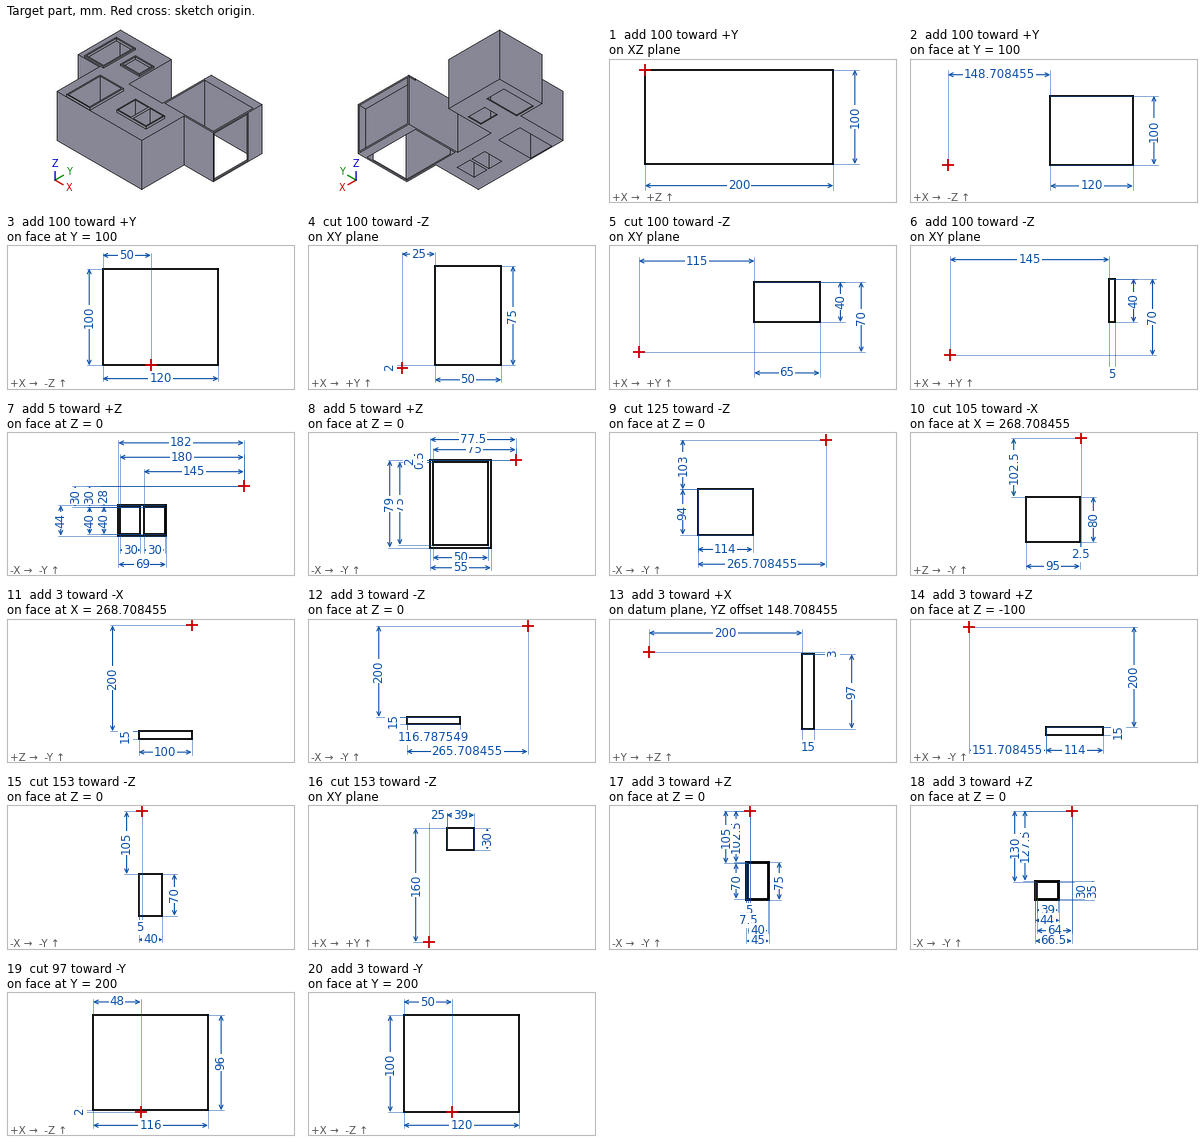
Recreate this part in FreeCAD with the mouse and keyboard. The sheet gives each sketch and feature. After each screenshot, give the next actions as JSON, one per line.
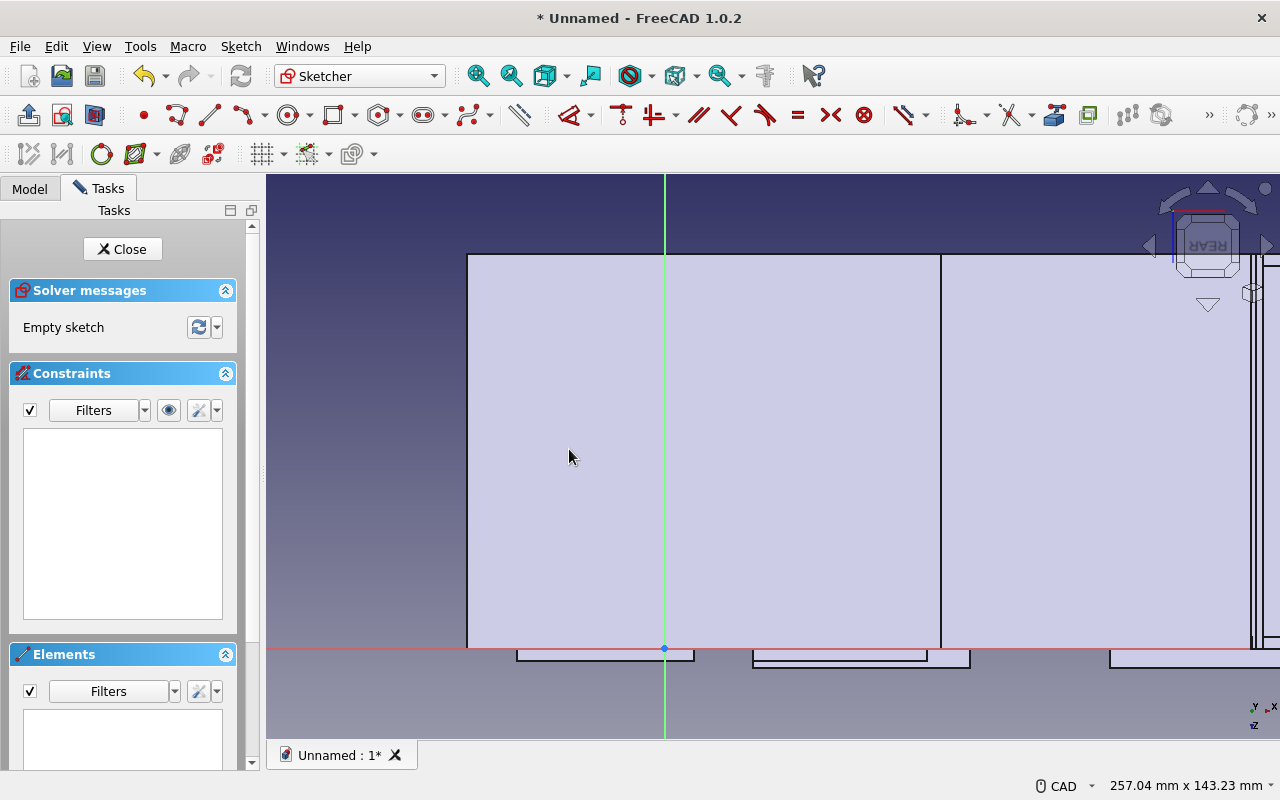
{"action": "left_click", "coordinate": [332, 116]}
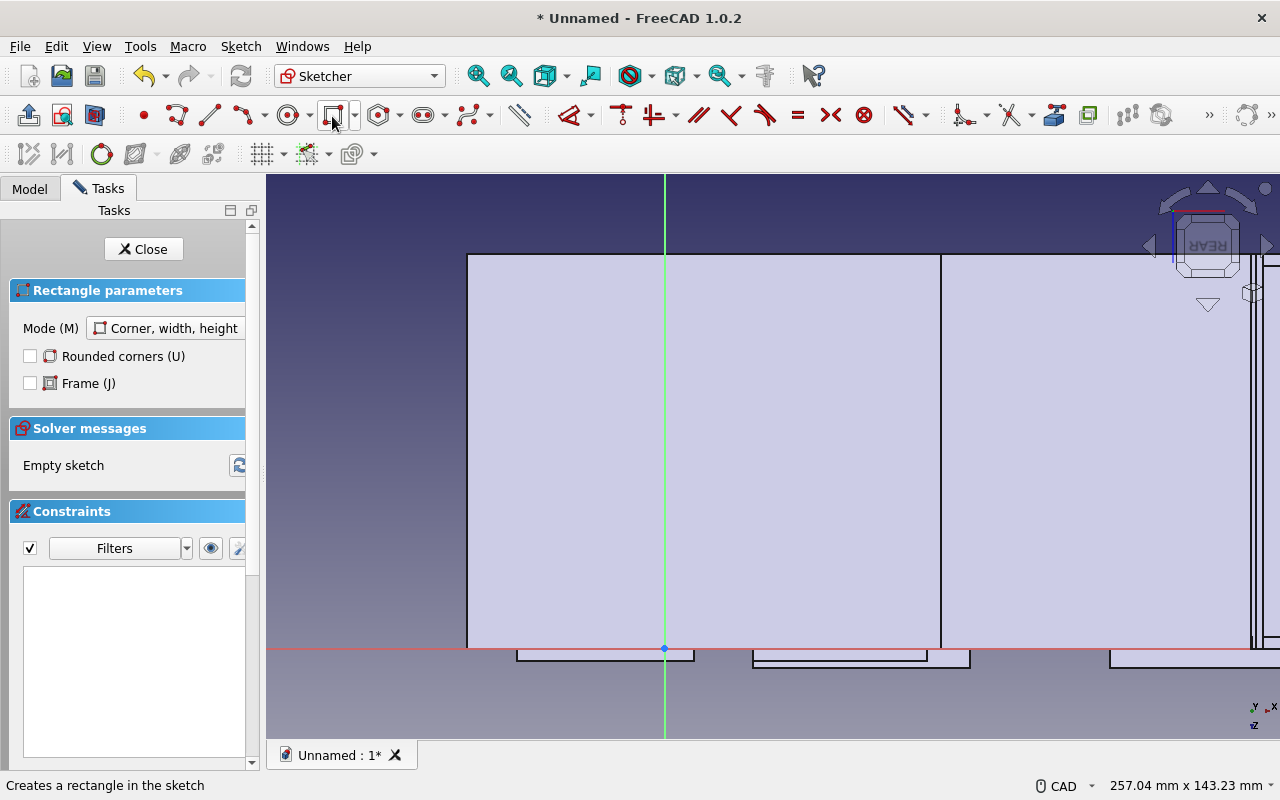
{"action": "left_click", "coordinate": [475, 262]}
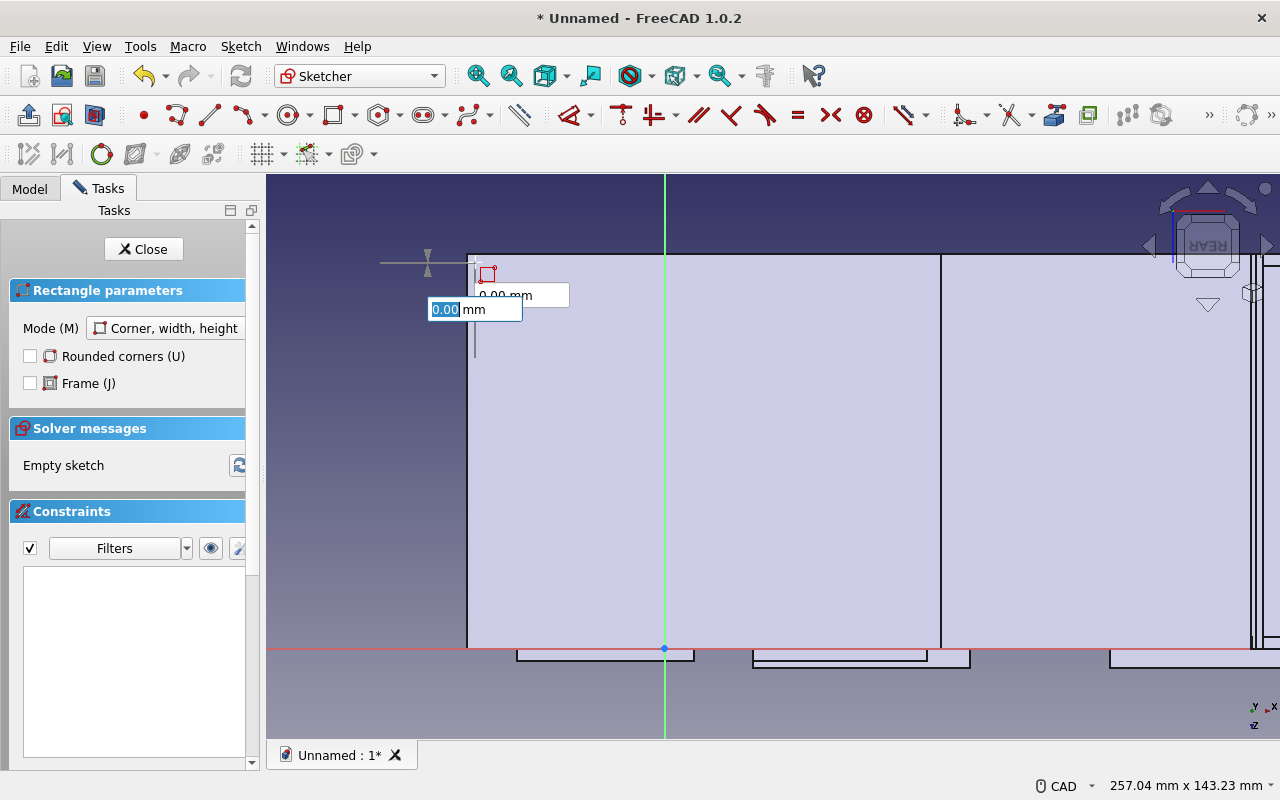
{"action": "scroll", "coordinate": [933, 641], "scroll_direction": "up", "scroll_amount": 4}
{"action": "mouse_move", "coordinate": [932, 640]}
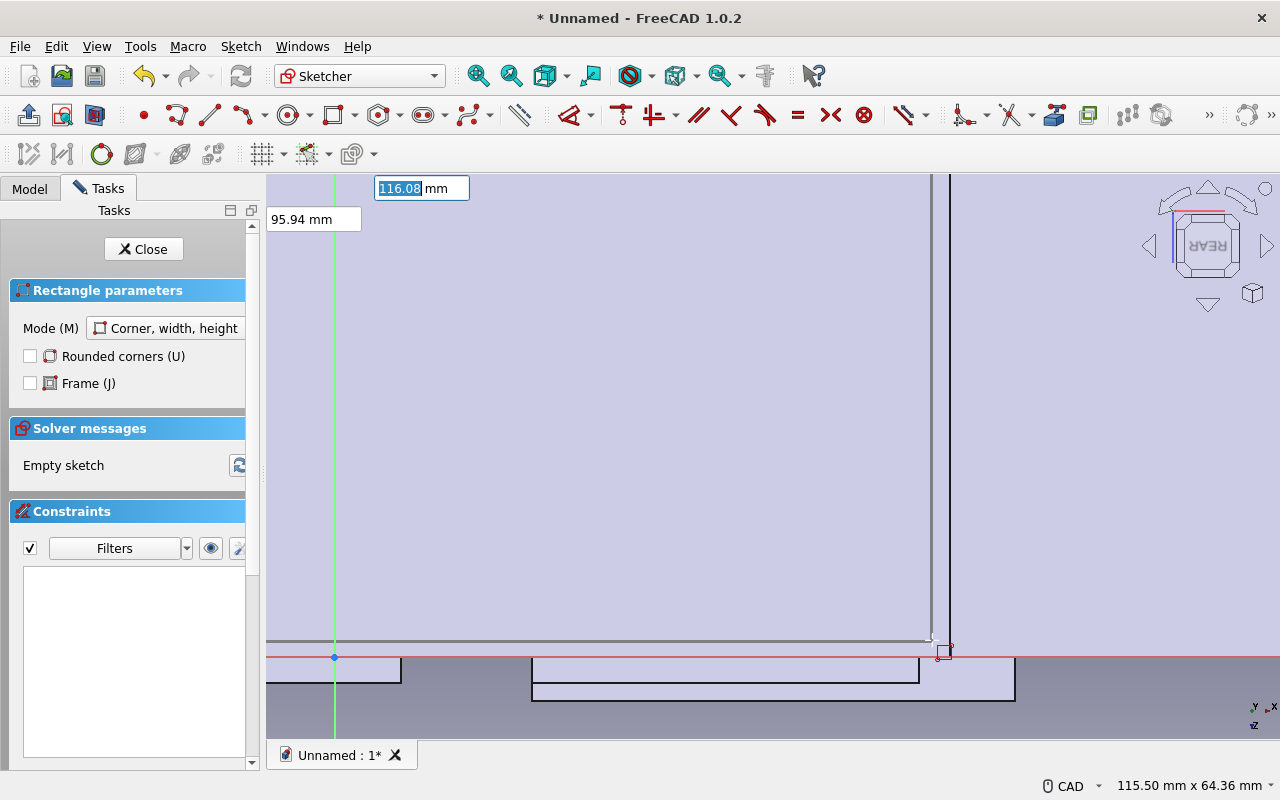
{"action": "type", "text": "116"}
{"action": "key", "text": "Tab"}
{"action": "type", "text": "96"}
{"action": "key", "text": "Return"}
{"action": "key", "text": "Escape"}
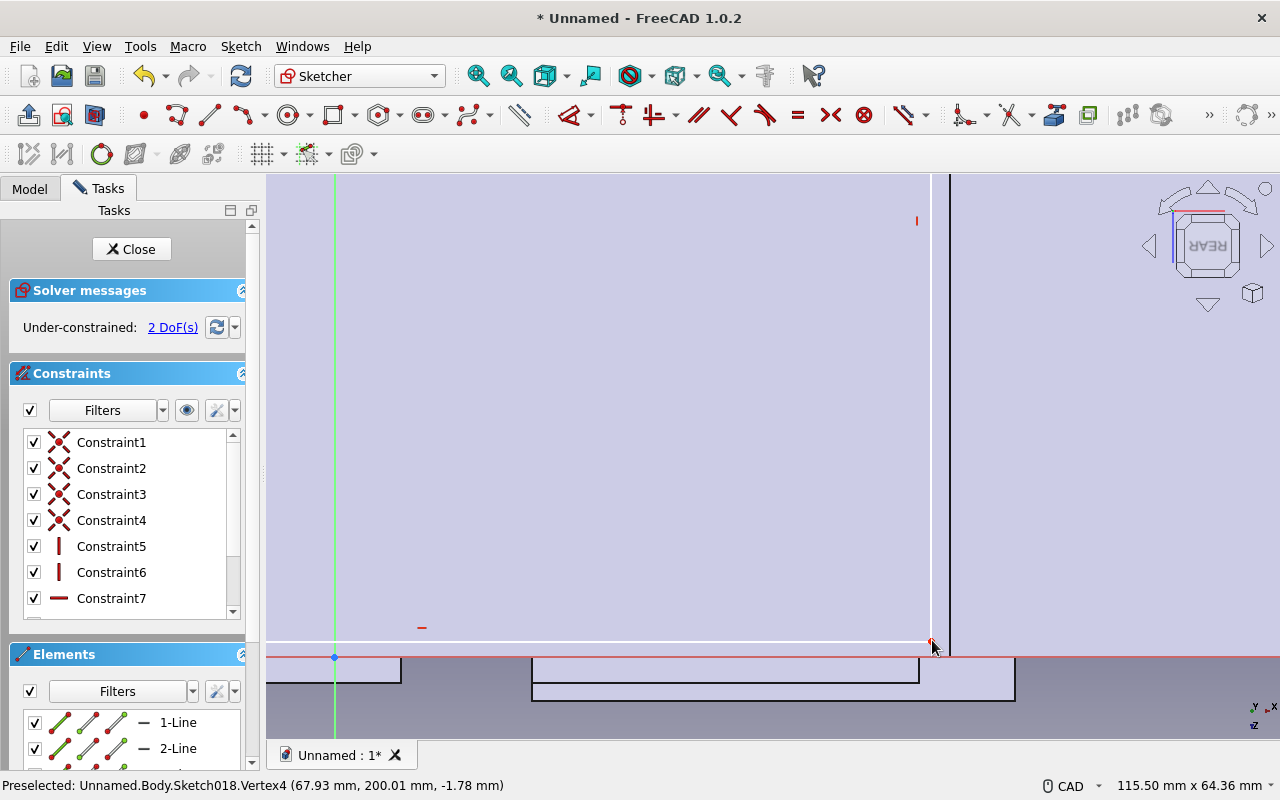
{"action": "left_click", "coordinate": [568, 116]}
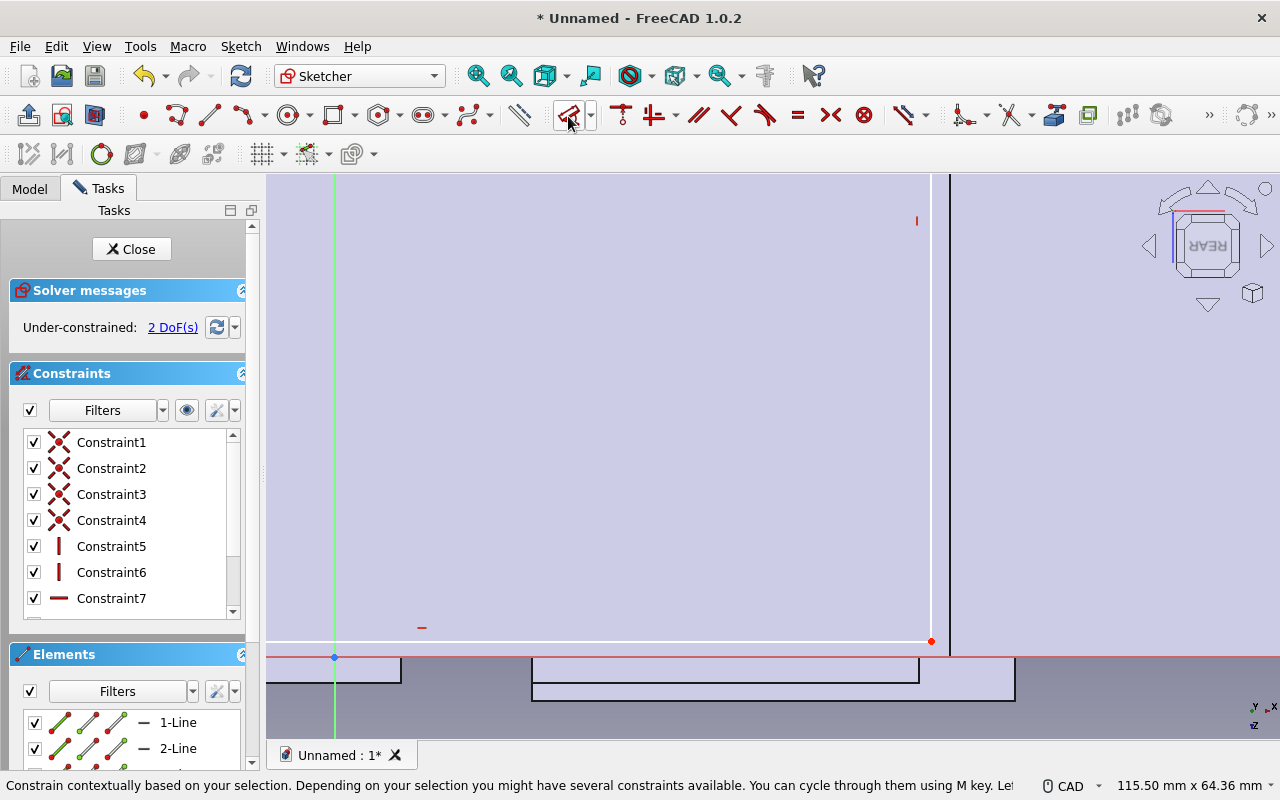
{"action": "scroll", "coordinate": [934, 644], "scroll_direction": "down", "scroll_amount": 4}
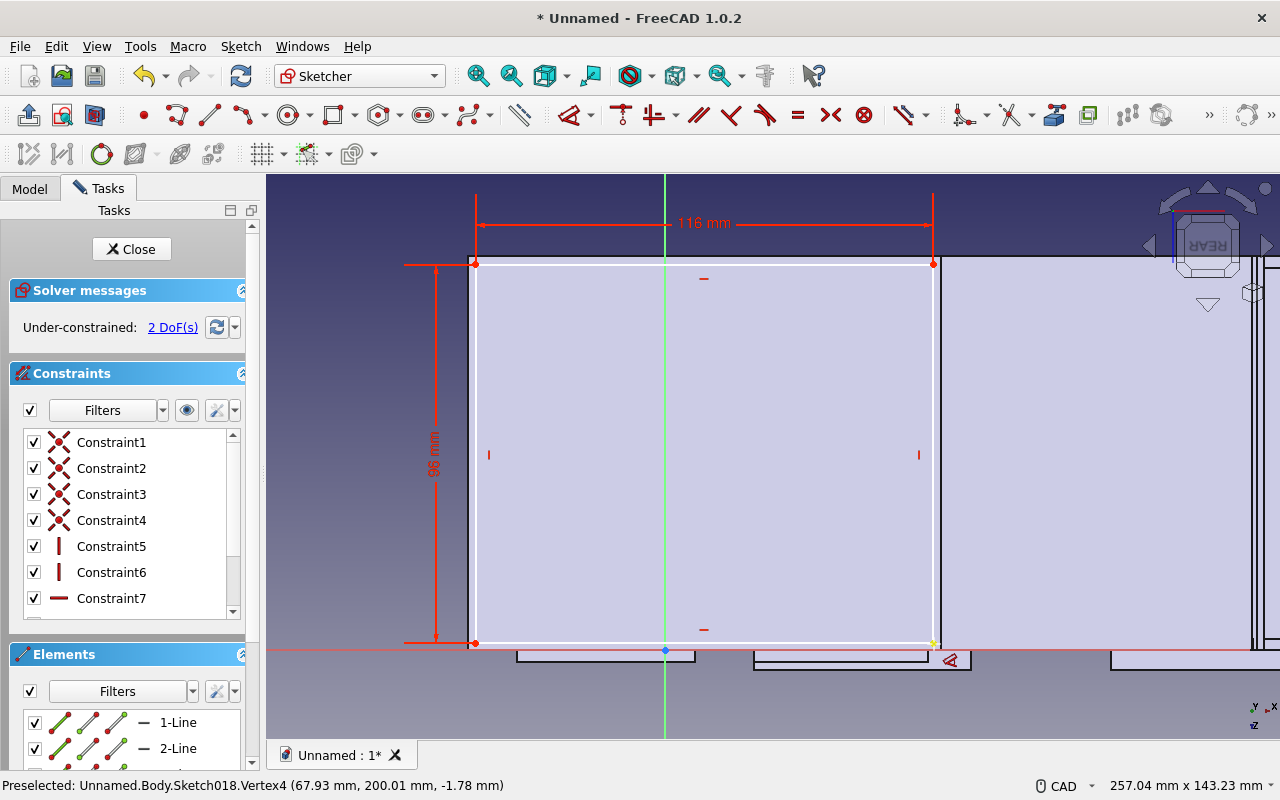
{"action": "scroll", "coordinate": [476, 643], "scroll_direction": "up", "scroll_amount": 9}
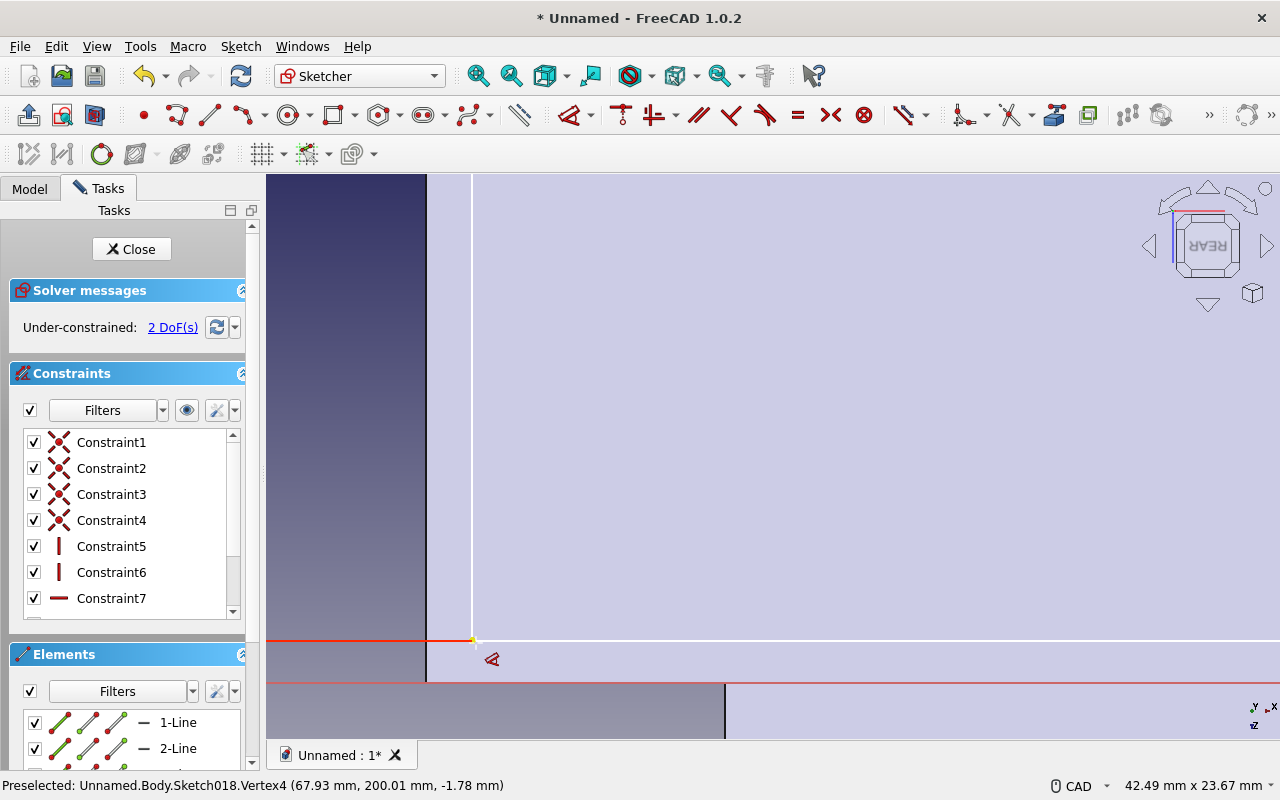
{"action": "left_click", "coordinate": [472, 641]}
{"action": "left_click", "coordinate": [438, 662]}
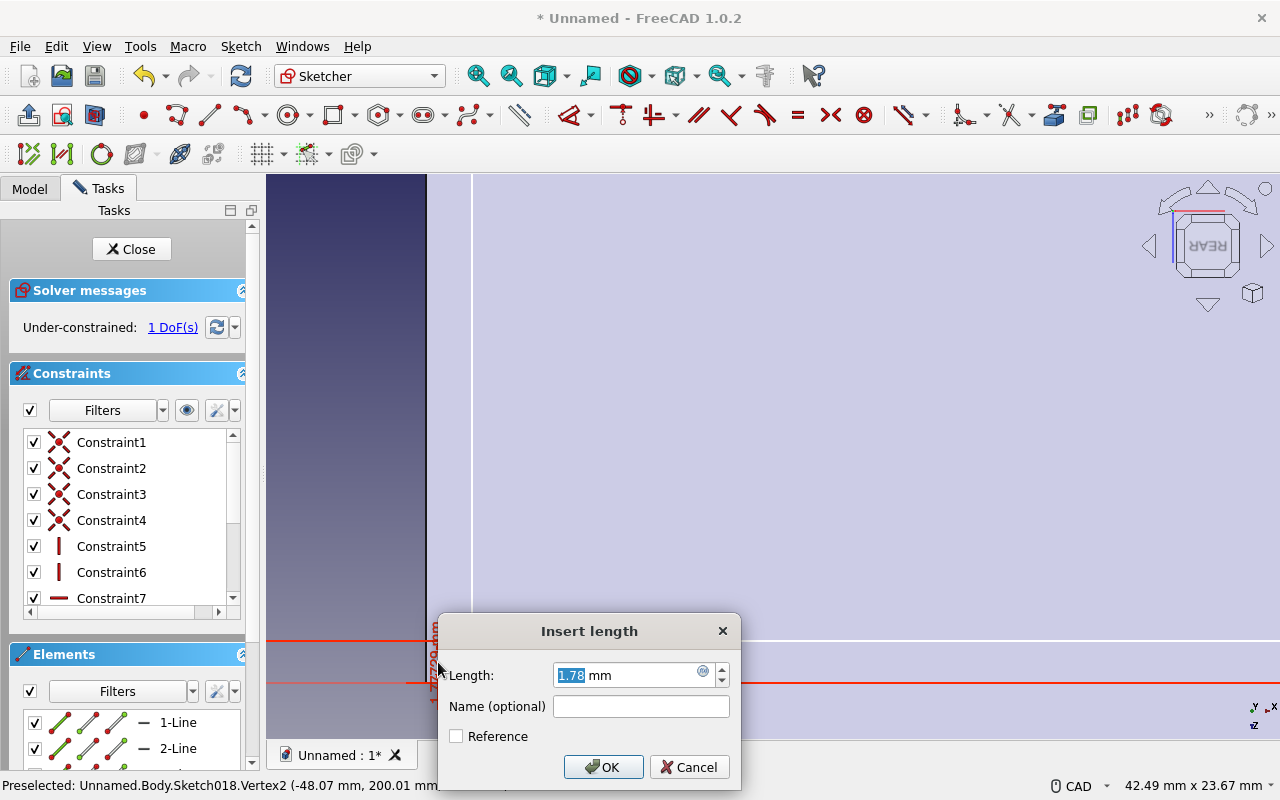
{"action": "type", "text": "2"}
{"action": "key", "text": "Return"}